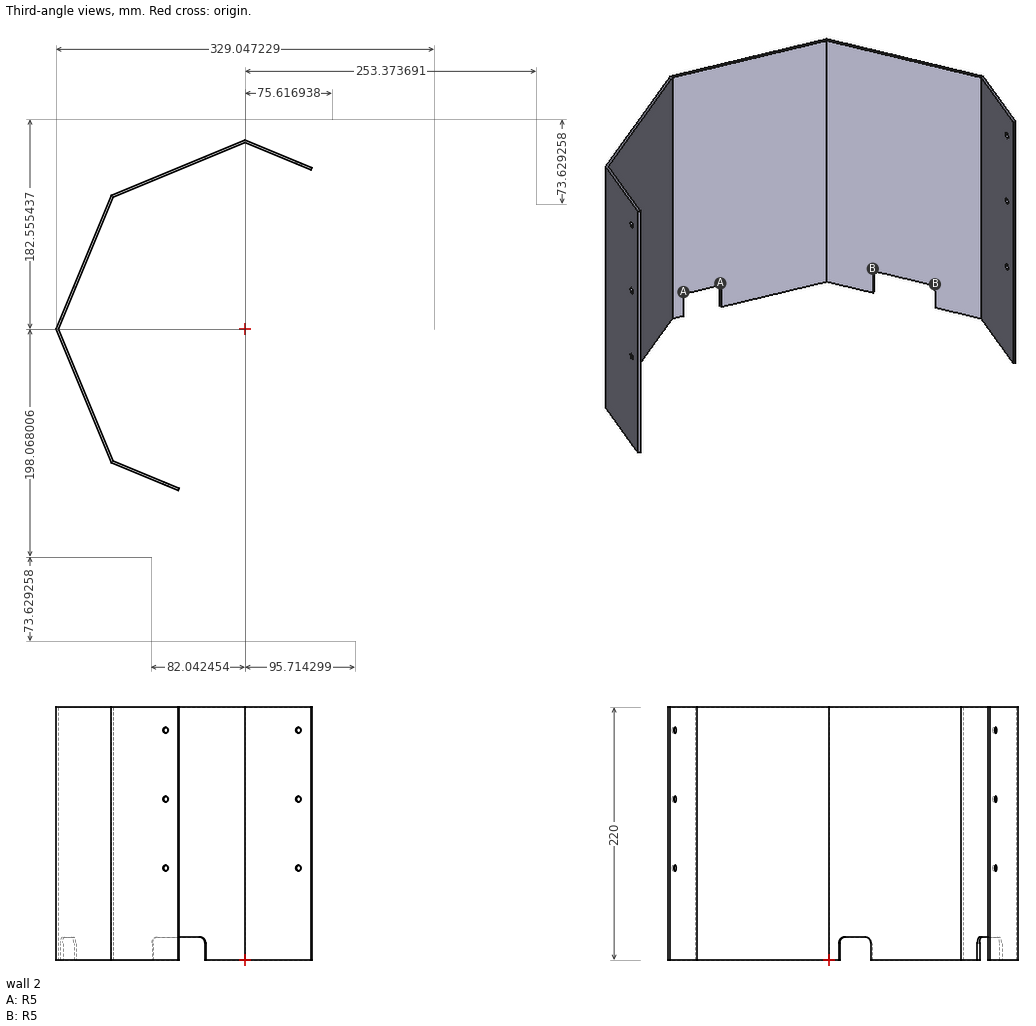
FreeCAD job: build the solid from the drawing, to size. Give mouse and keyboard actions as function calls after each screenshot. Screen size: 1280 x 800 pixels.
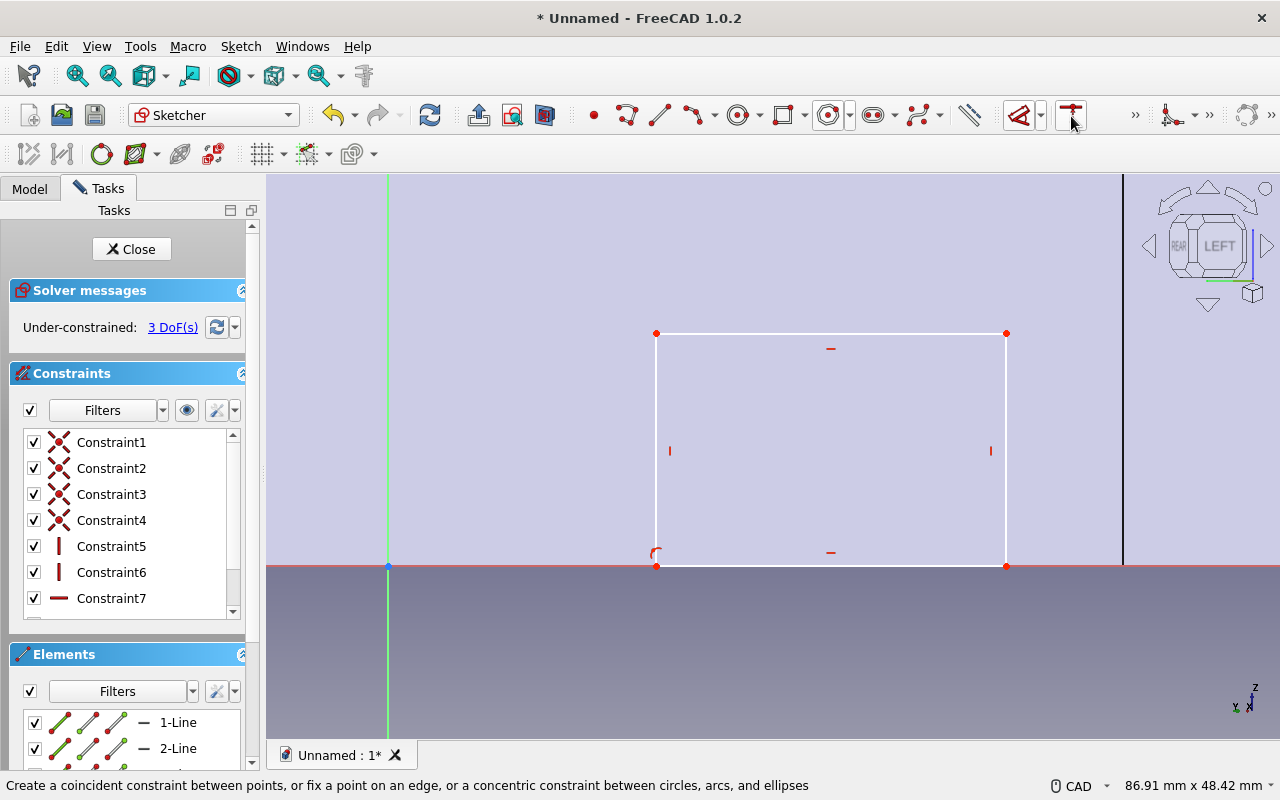
click(656, 404)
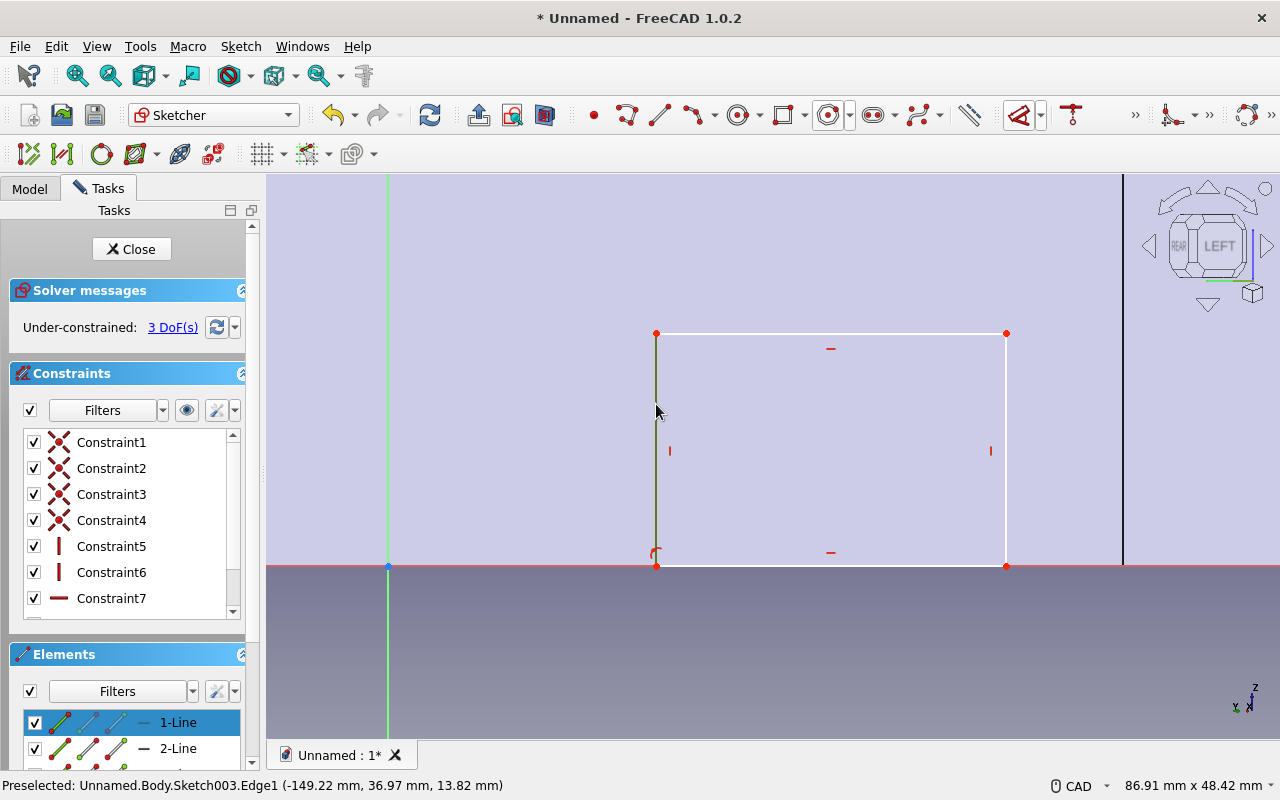
click(1040, 116)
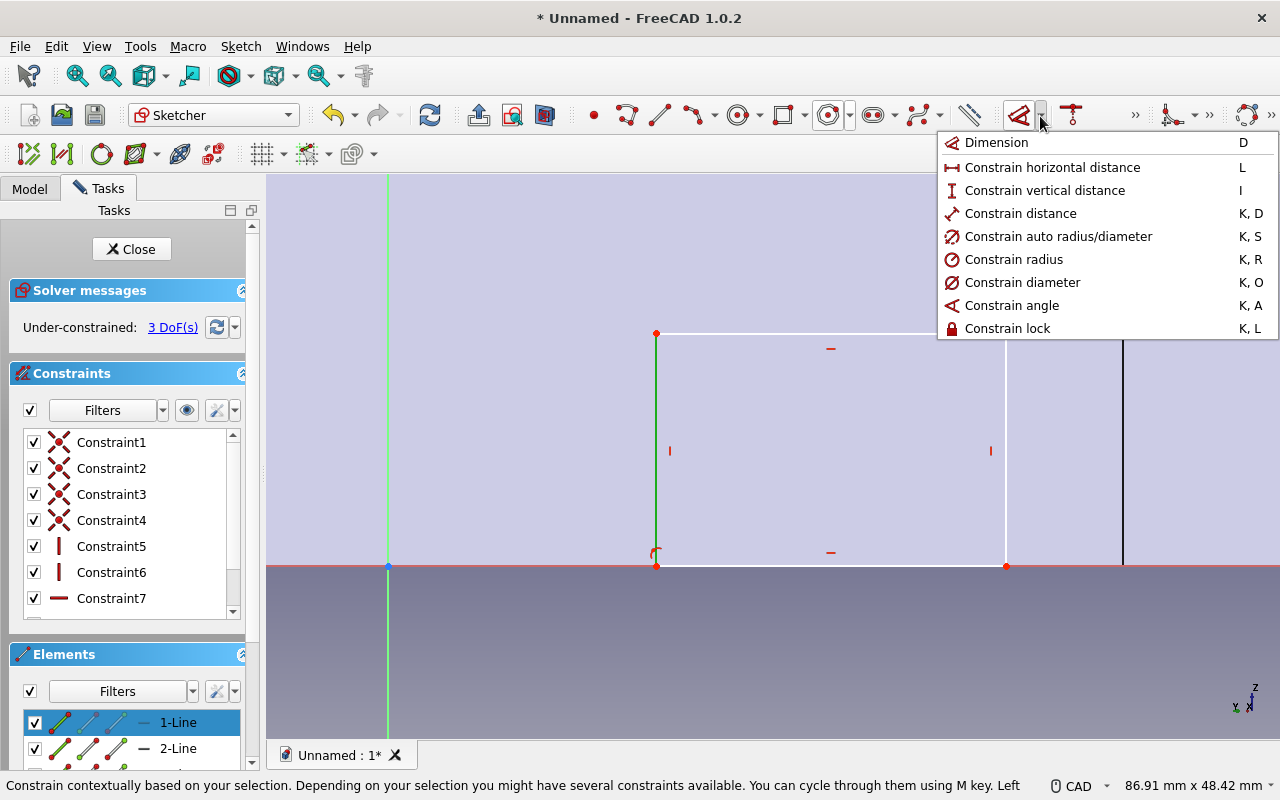
click(1108, 190)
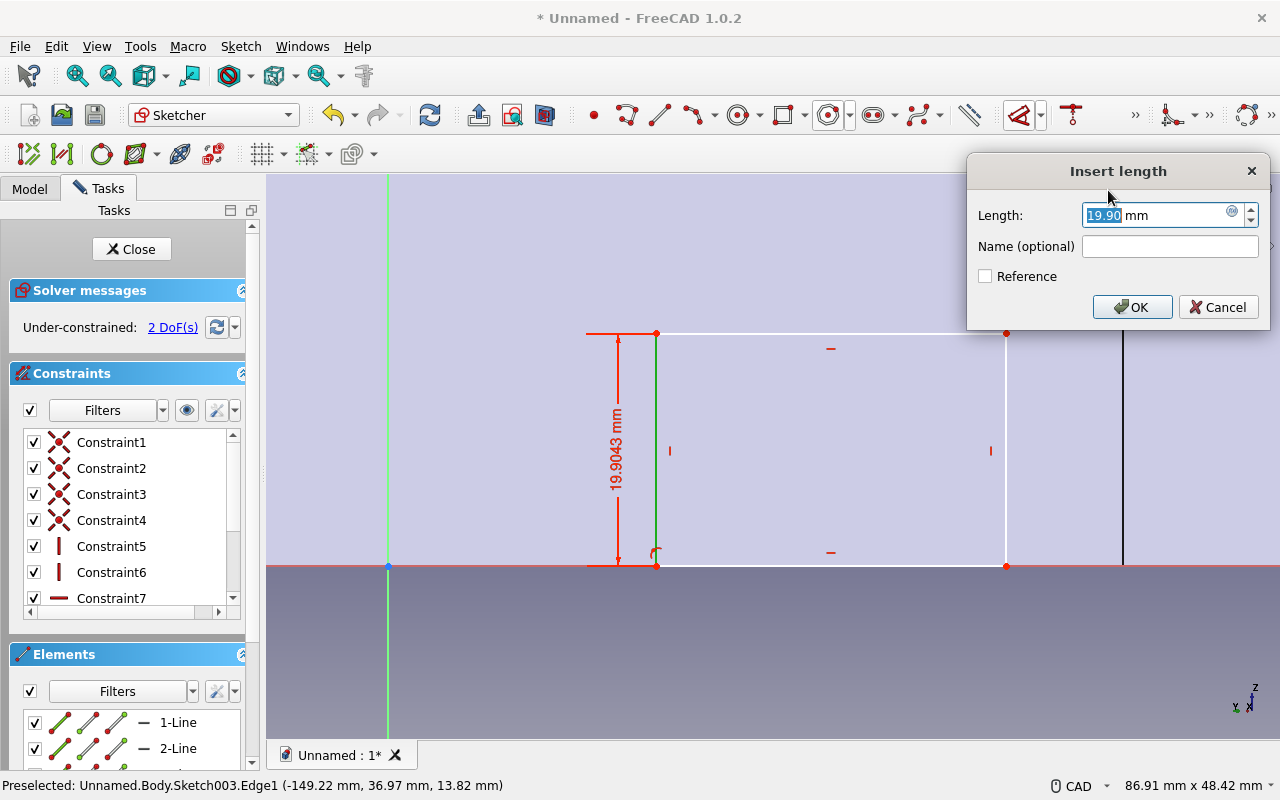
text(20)
key(Return)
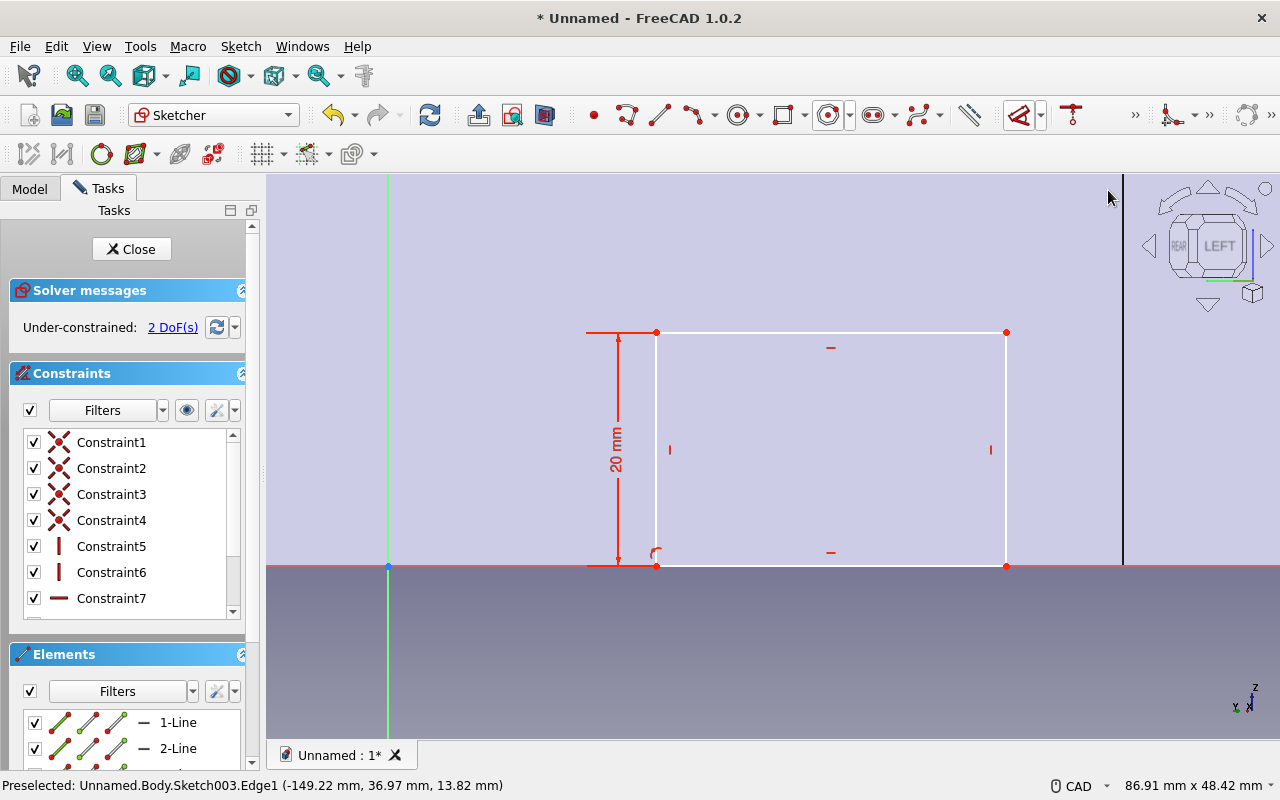
click(761, 566)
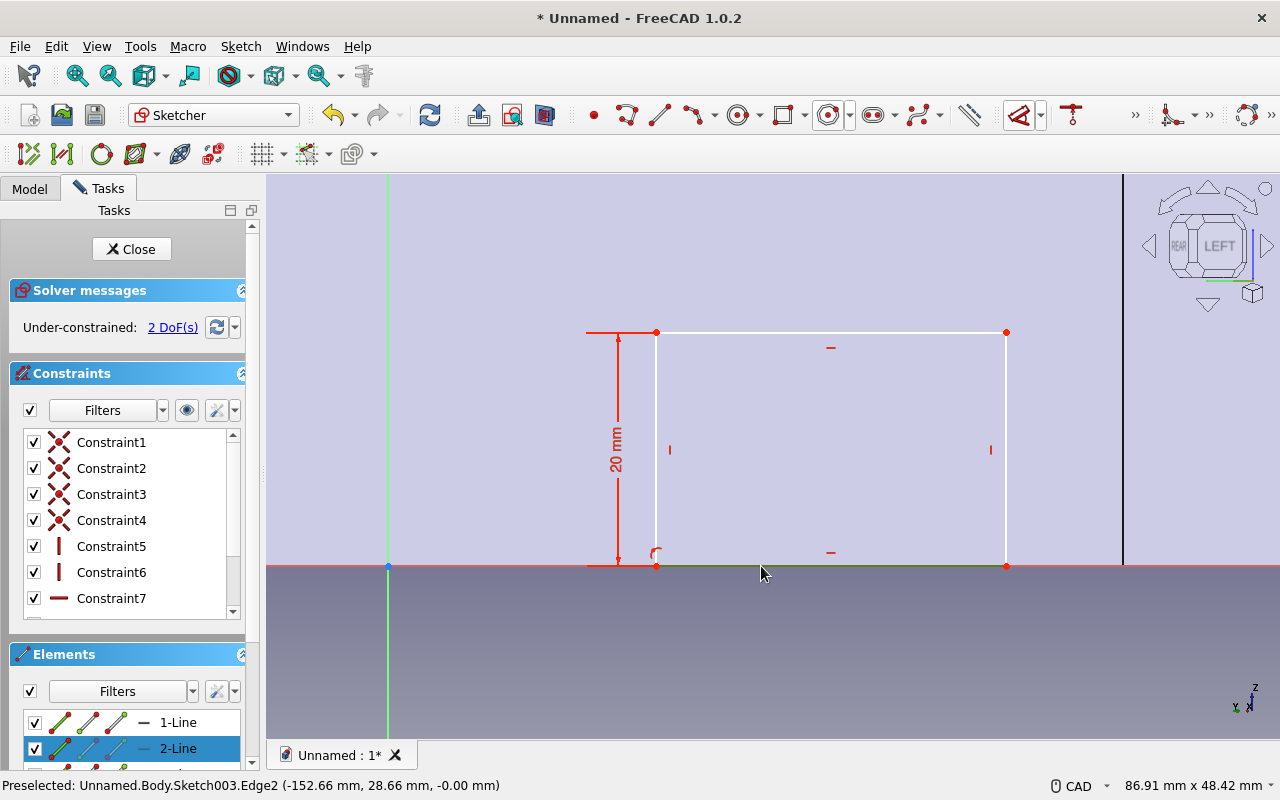
click(1040, 116)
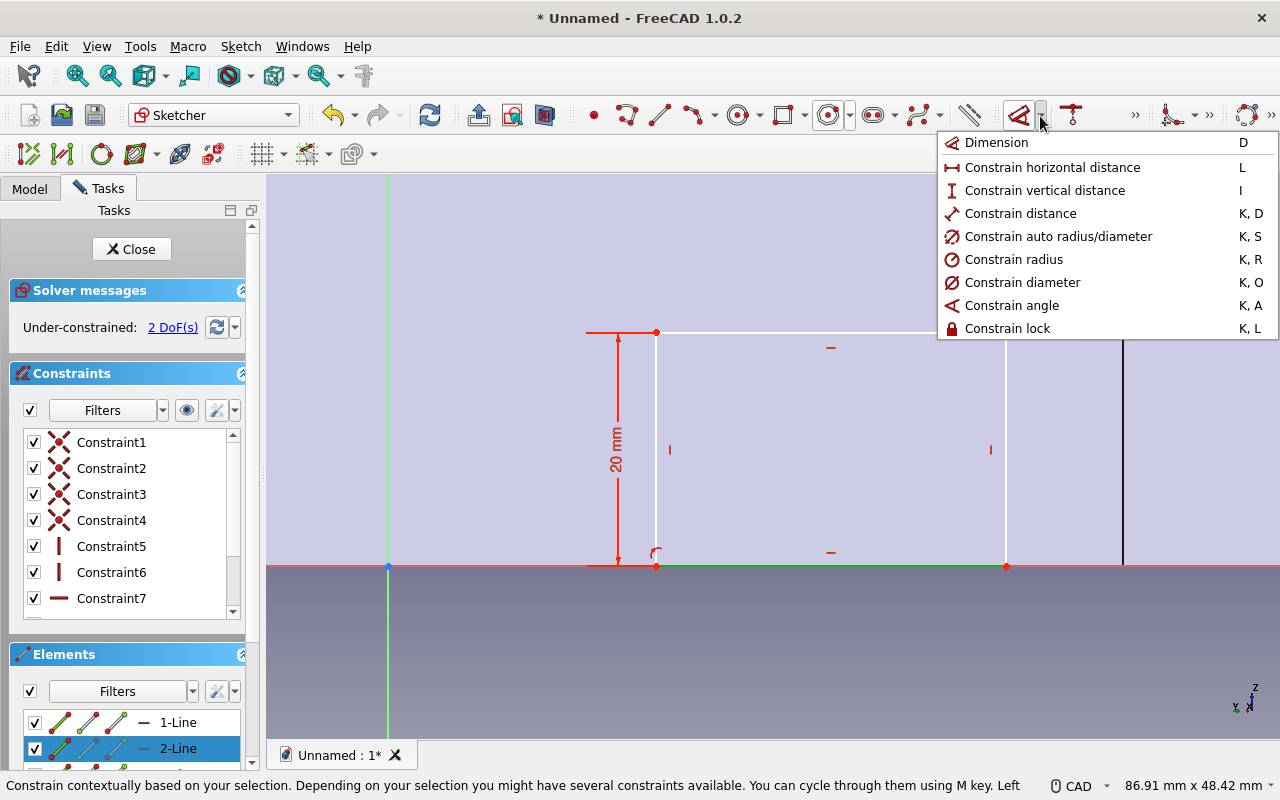
click(1108, 168)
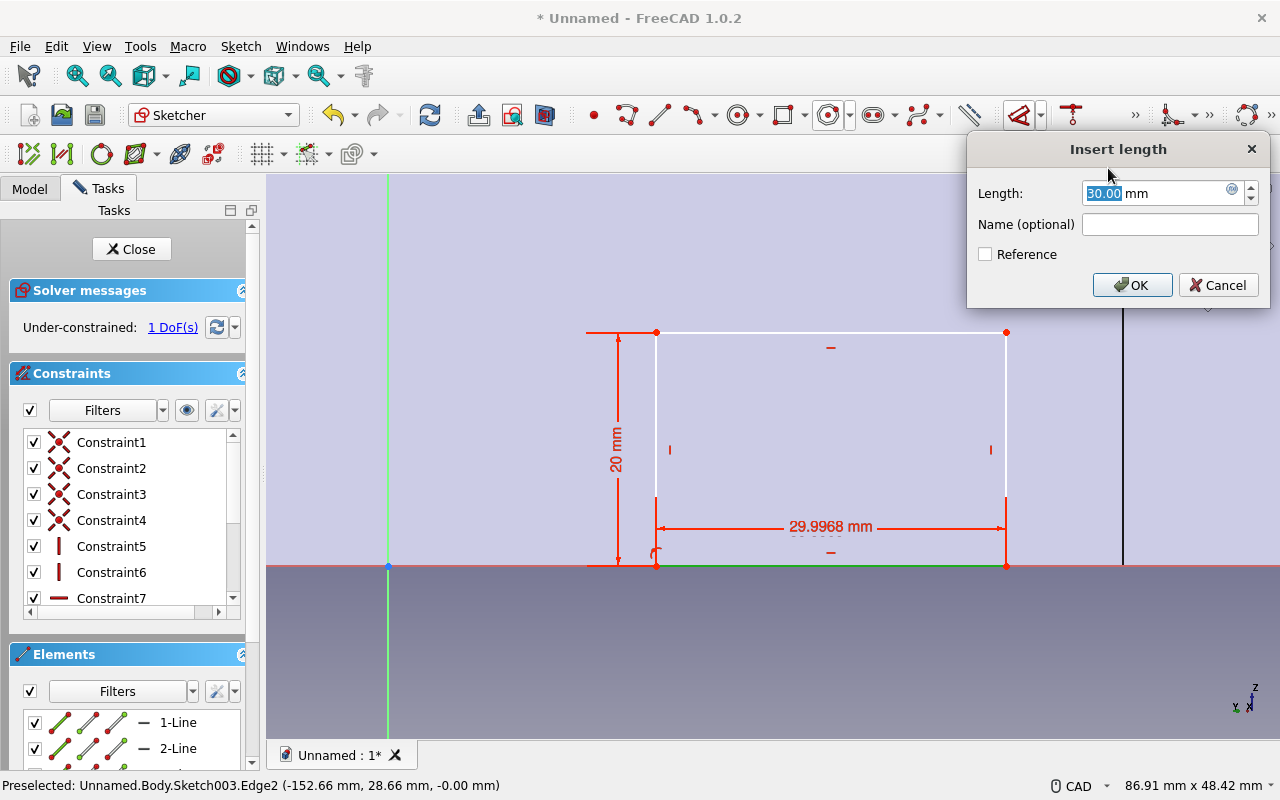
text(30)
key(Return)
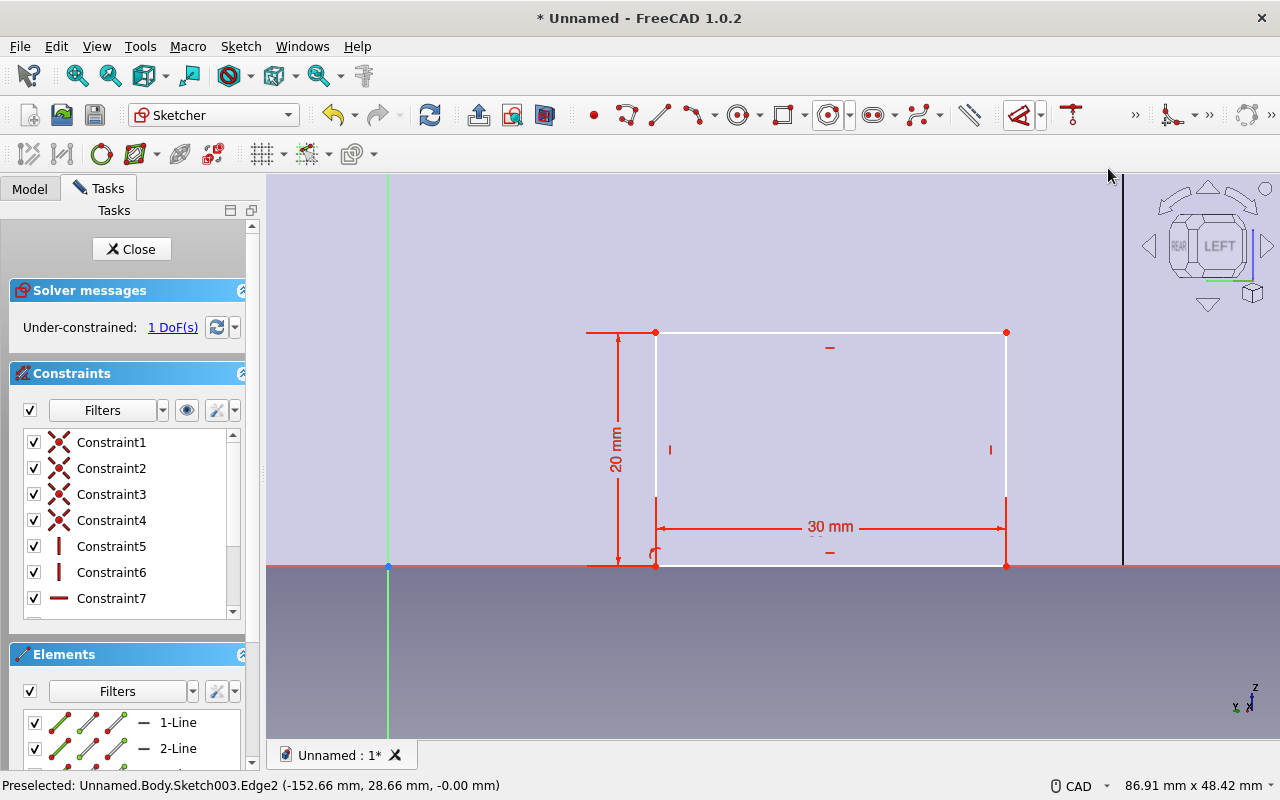
click(656, 333)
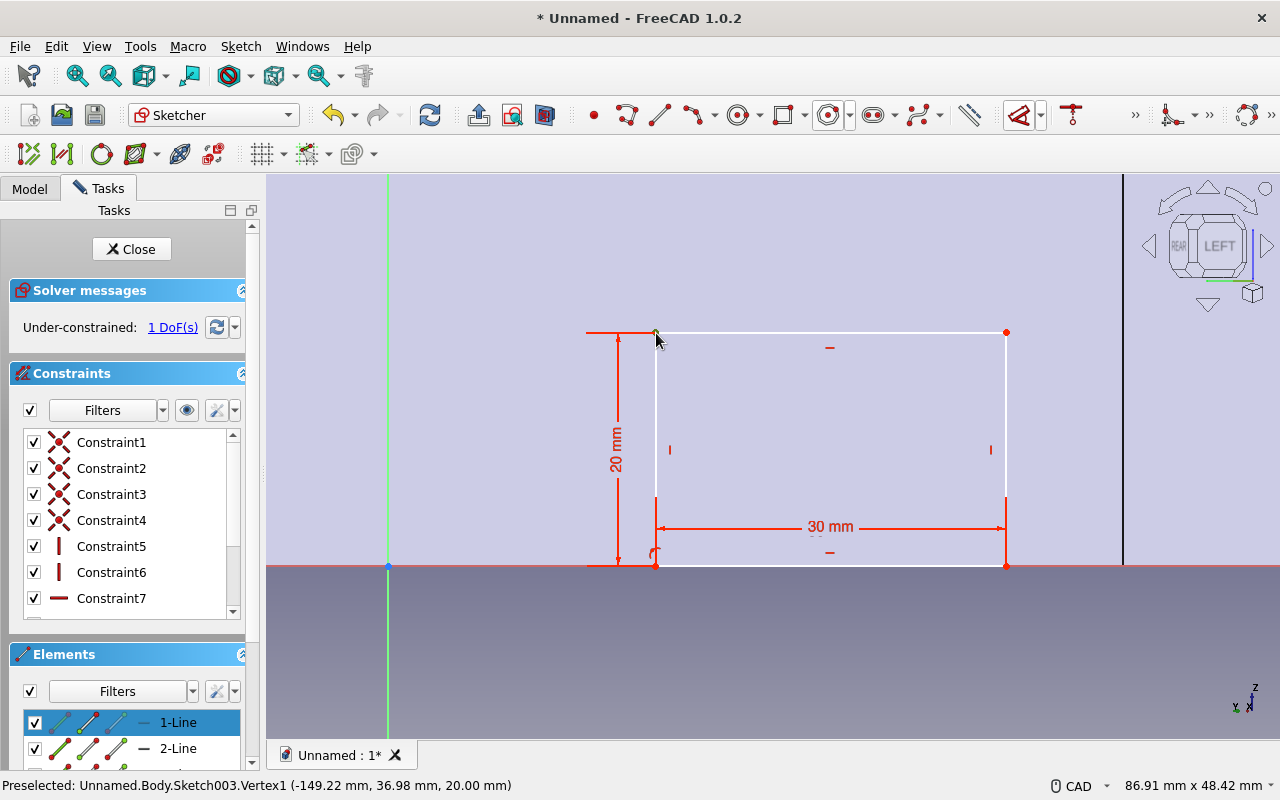
click(1040, 116)